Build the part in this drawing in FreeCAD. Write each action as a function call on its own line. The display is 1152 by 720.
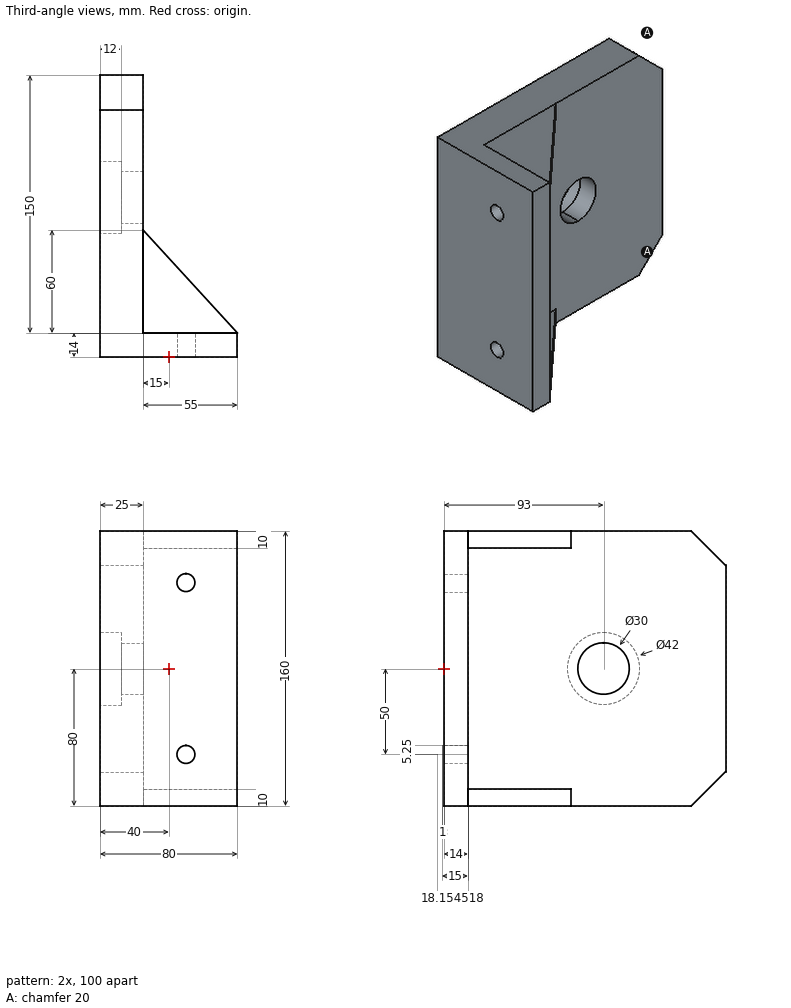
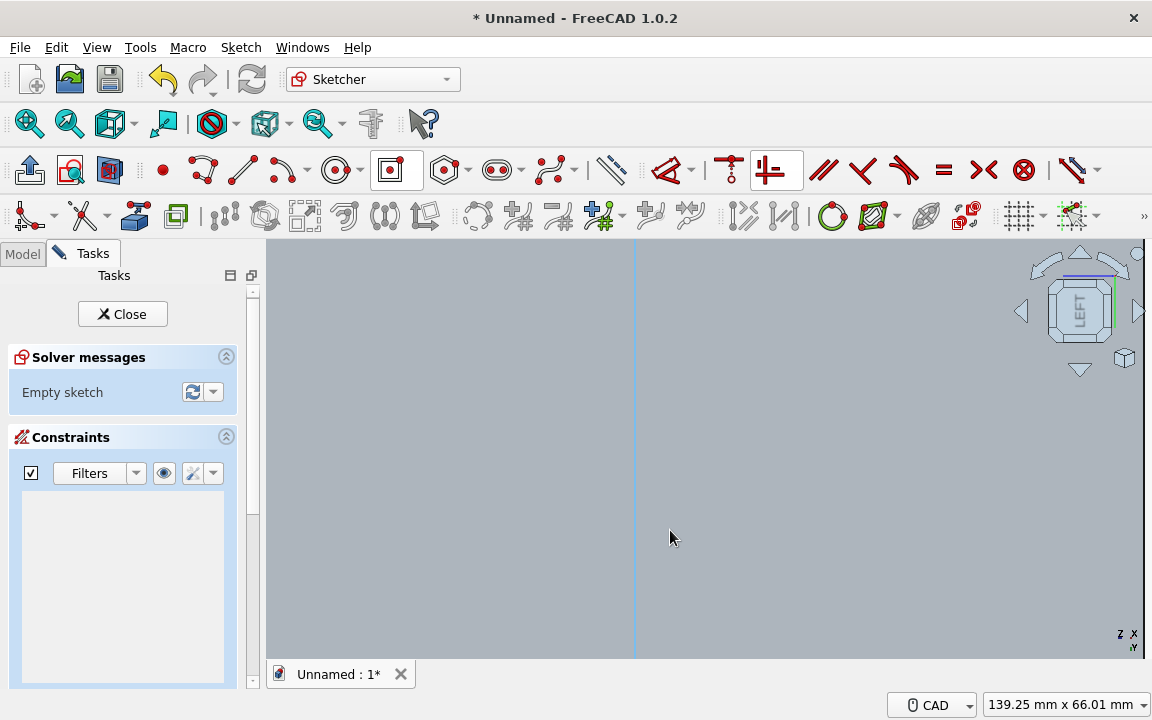
key(g)
key(c)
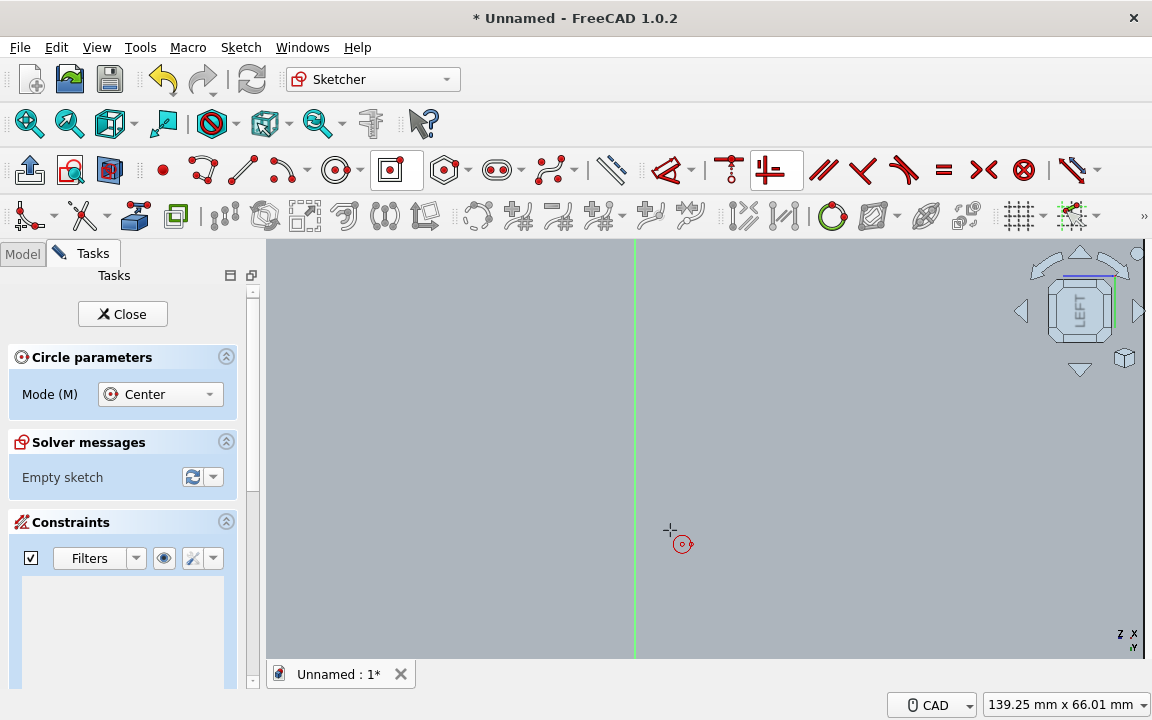
click(635, 445)
move(729, 350)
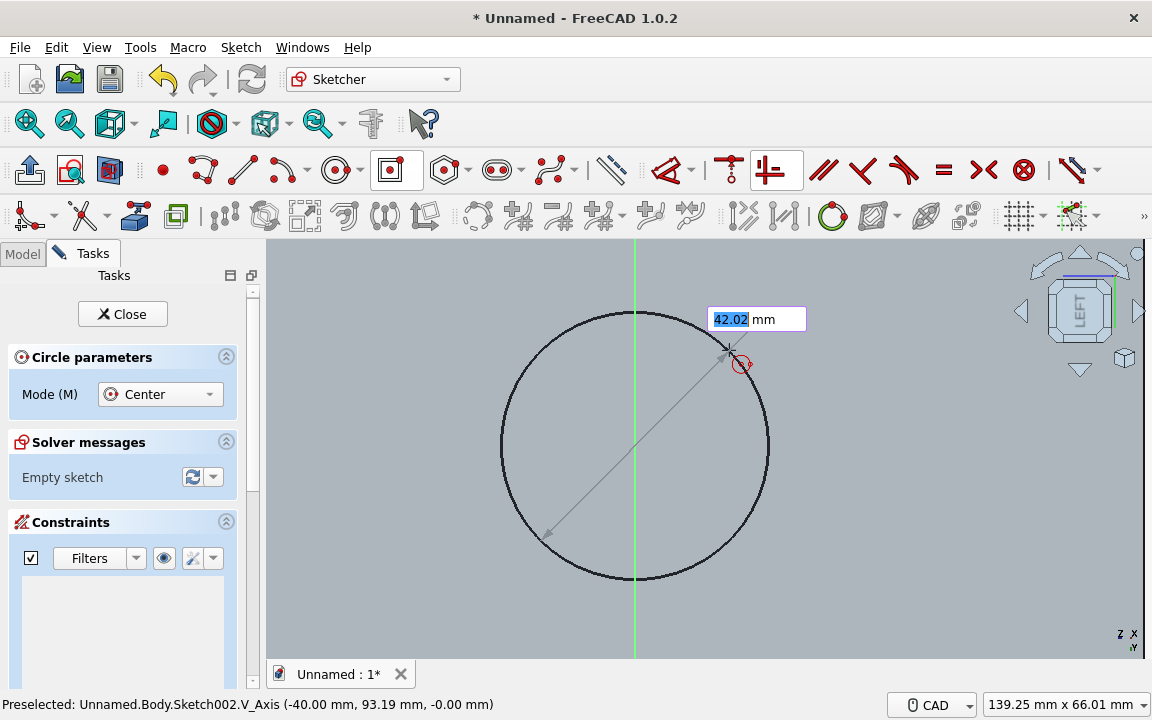
text(42)
key(Return)
key(Escape)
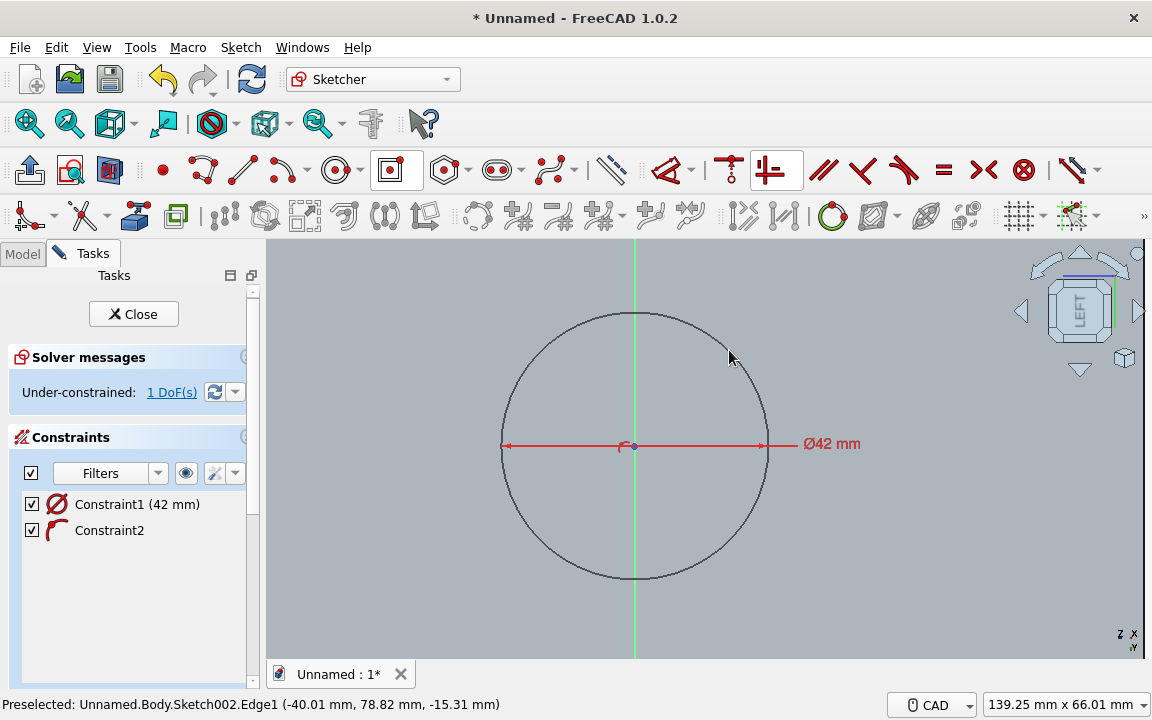
click(666, 170)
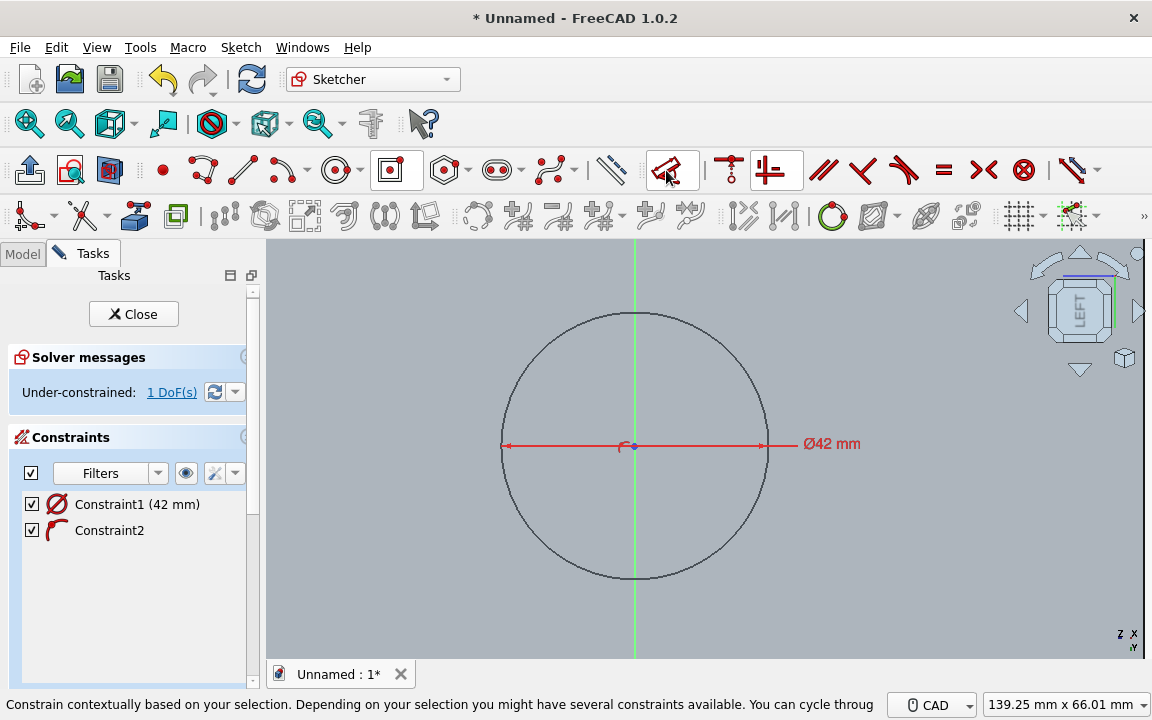
click(635, 446)
click(669, 357)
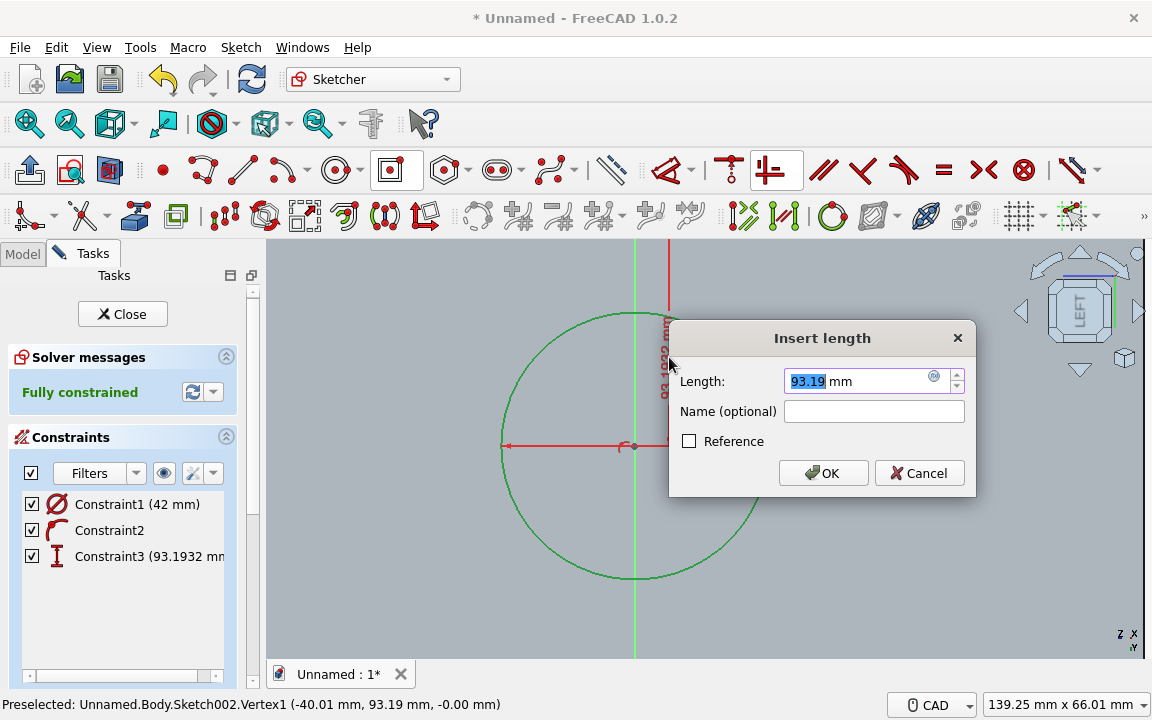
text(93)
key(Return)
key(Escape)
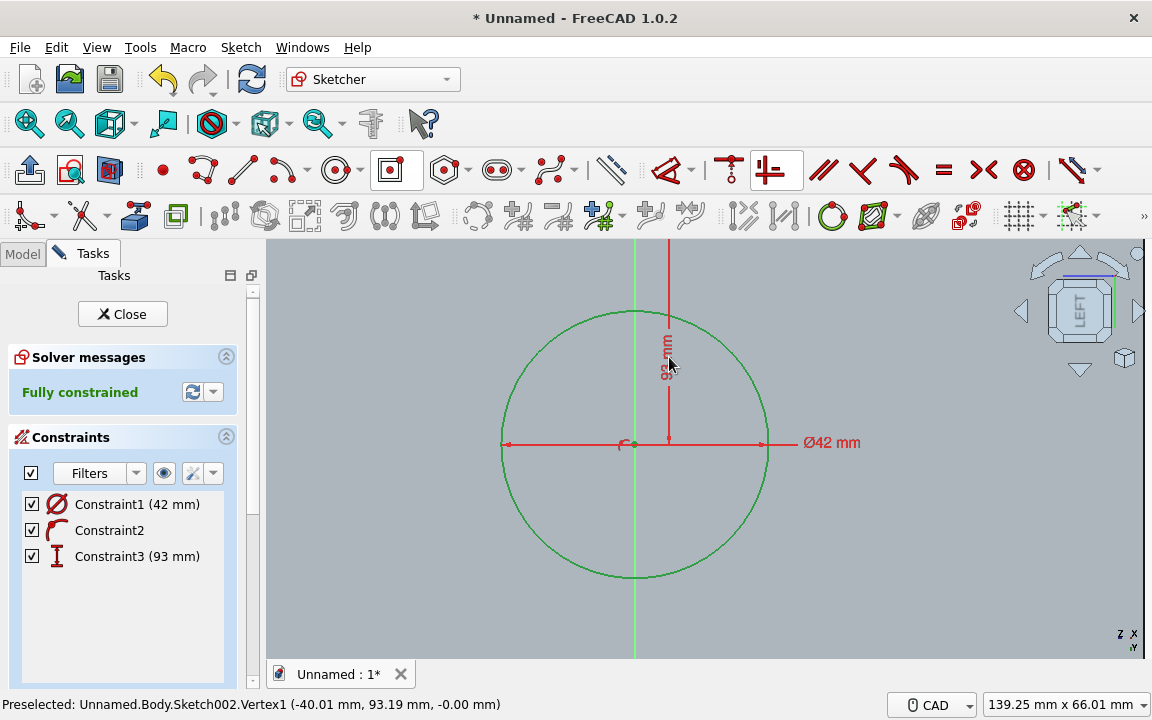
click(123, 314)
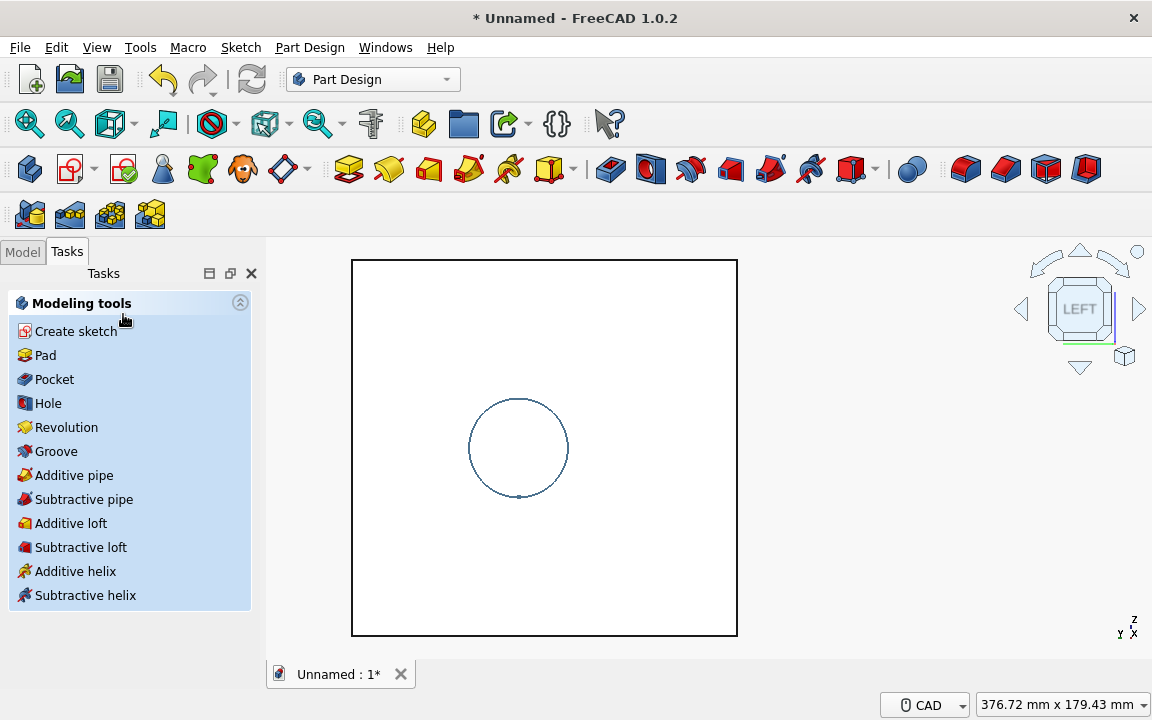
click(612, 170)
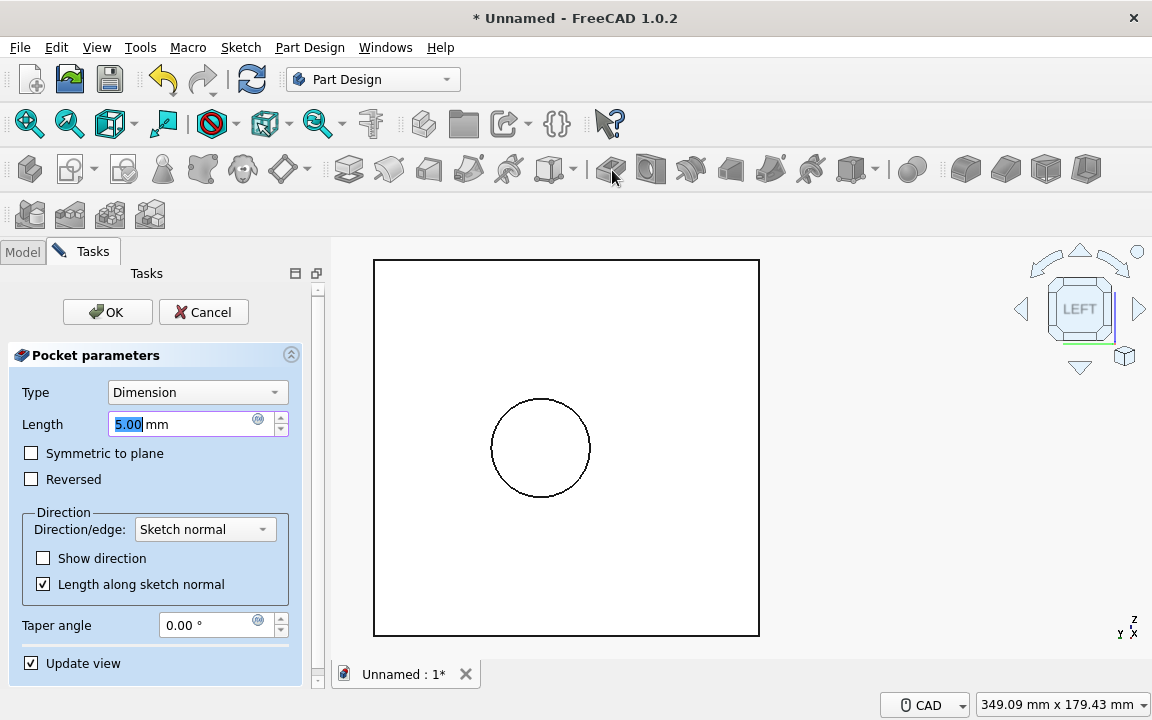
text(12)
key(Tab)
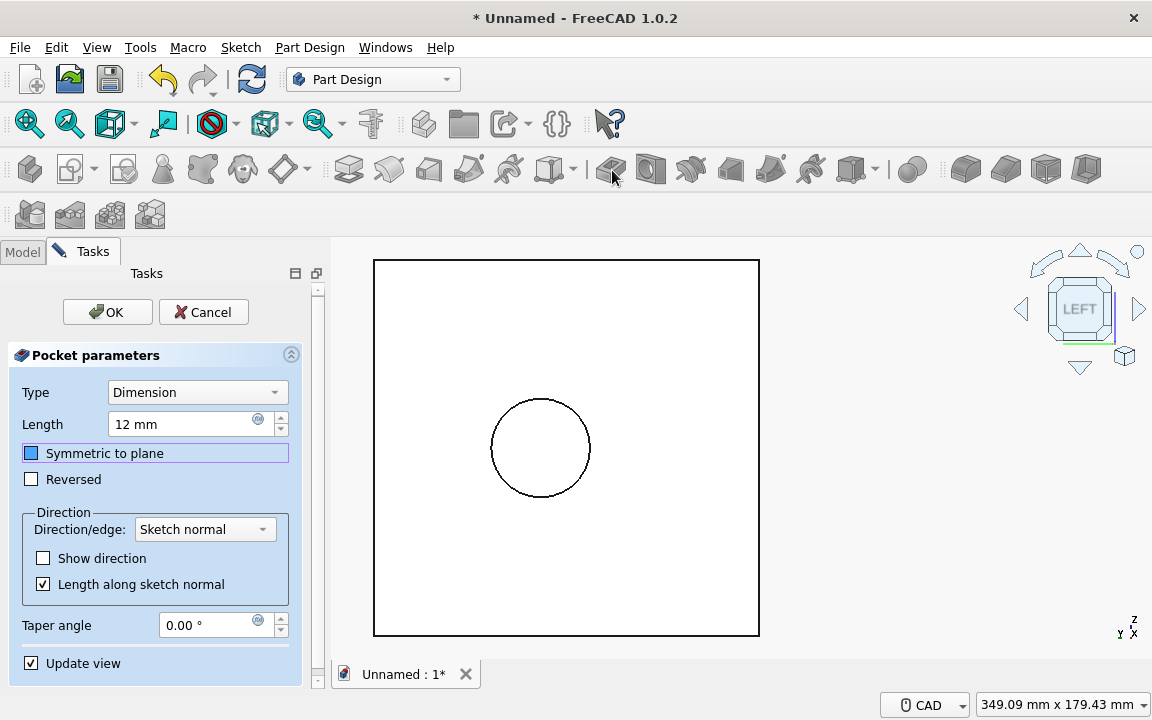
click(108, 312)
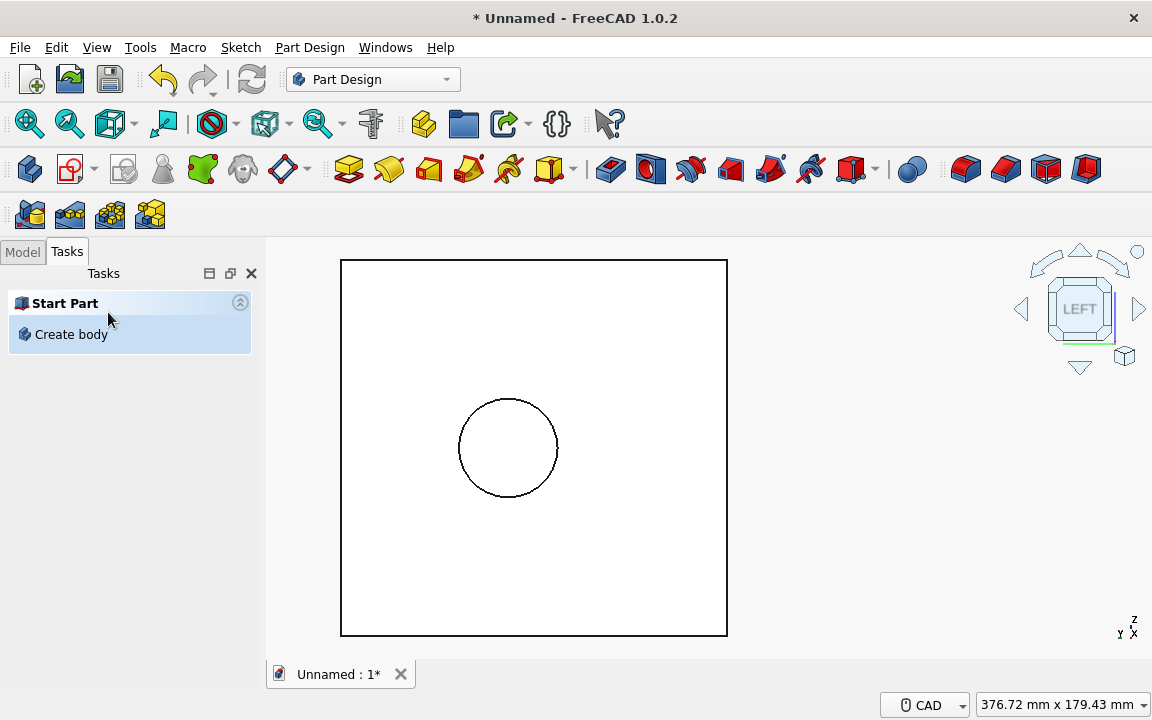
click(508, 447)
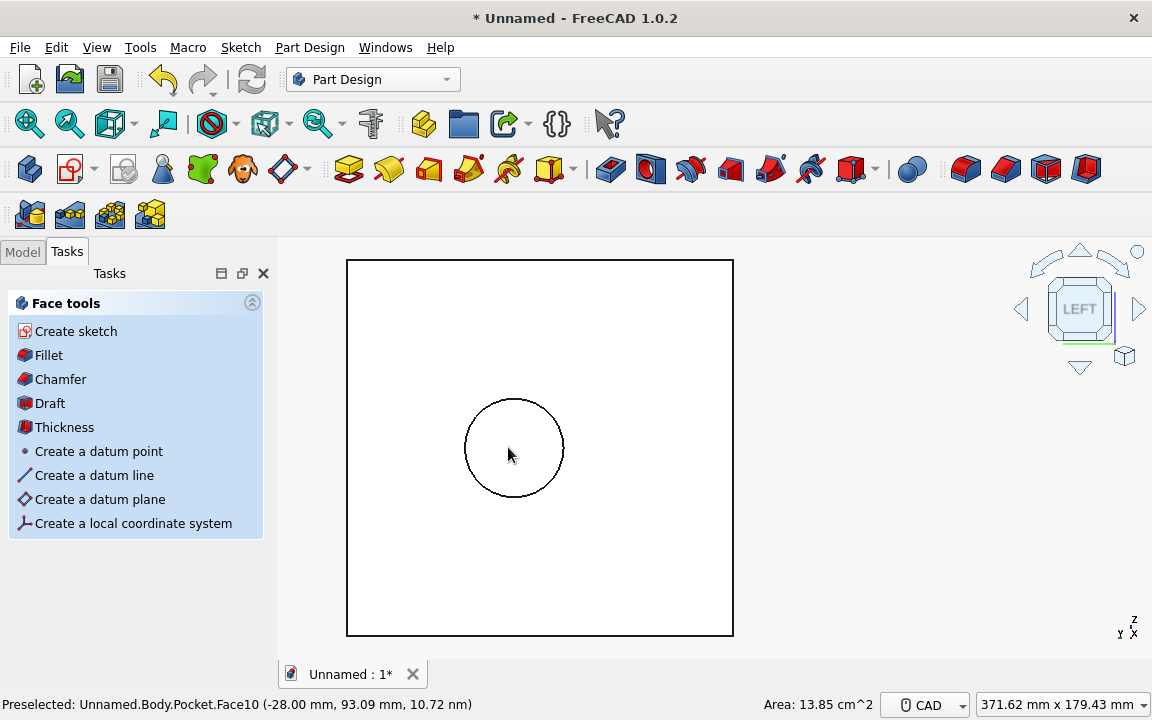
click(70, 170)